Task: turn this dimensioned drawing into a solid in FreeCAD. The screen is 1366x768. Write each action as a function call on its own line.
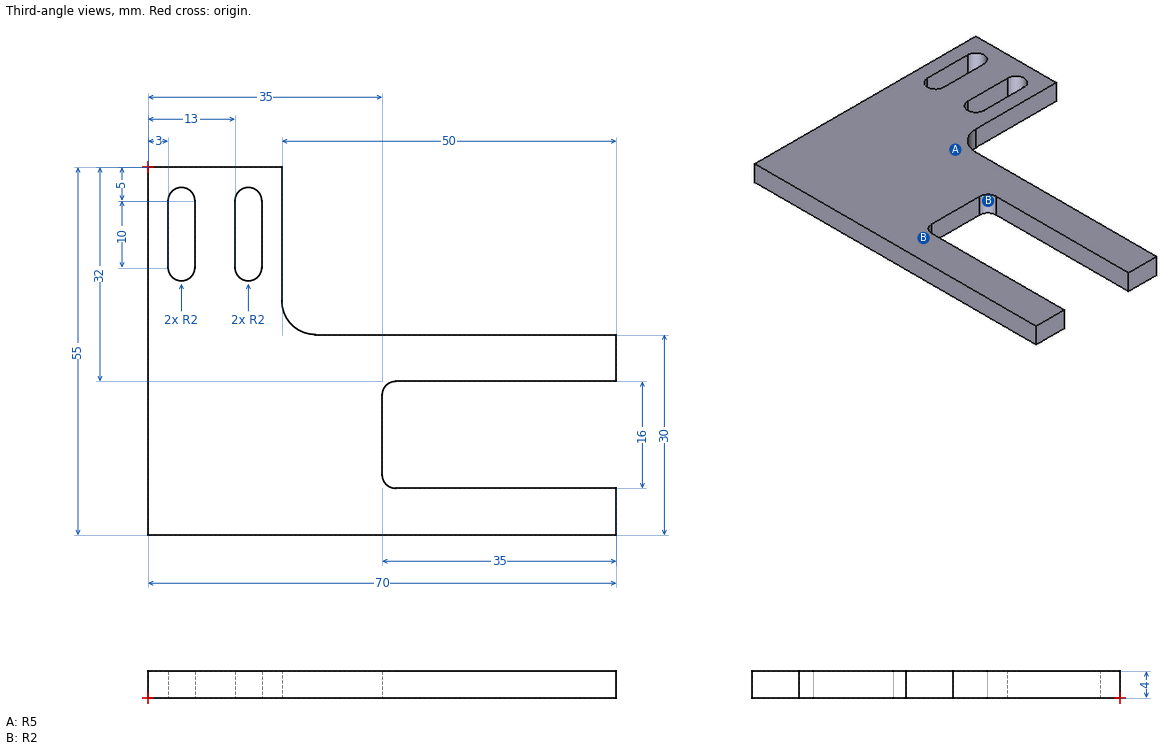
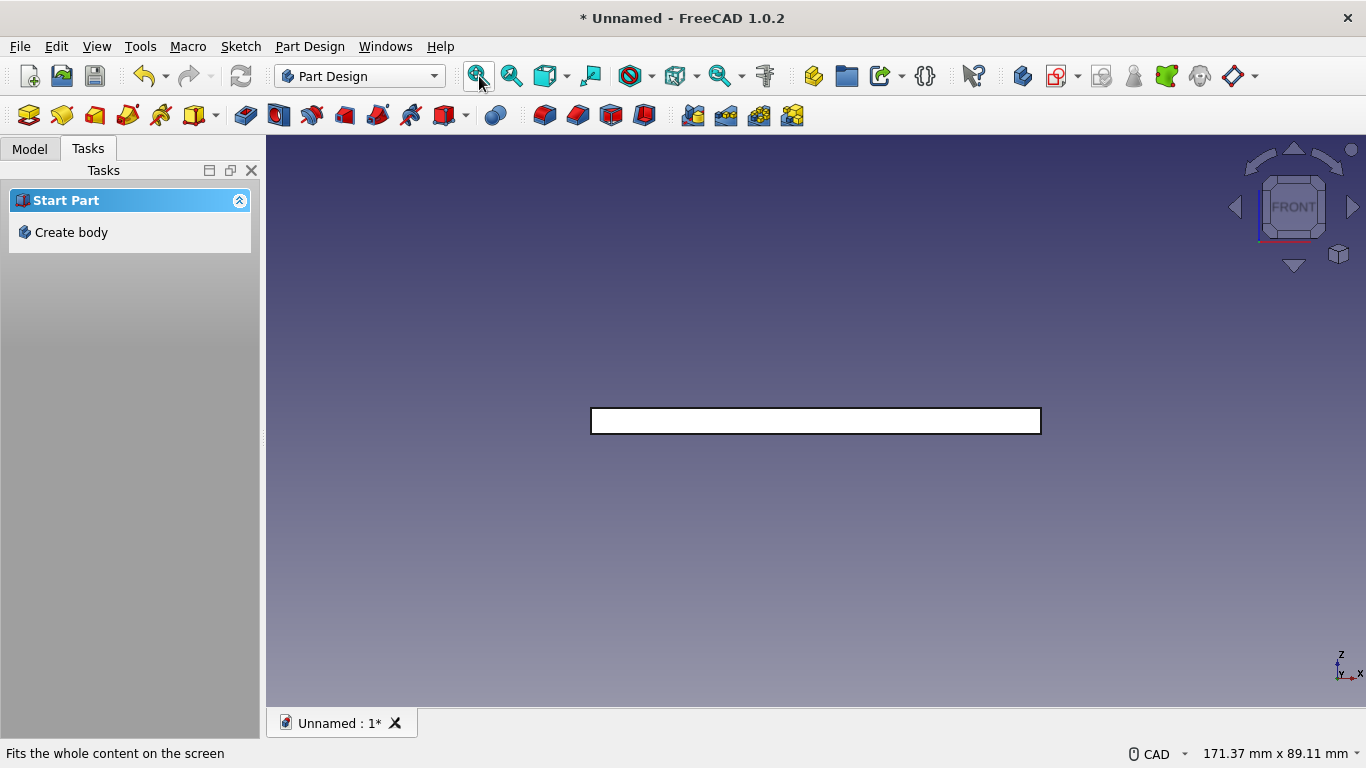
click(479, 76)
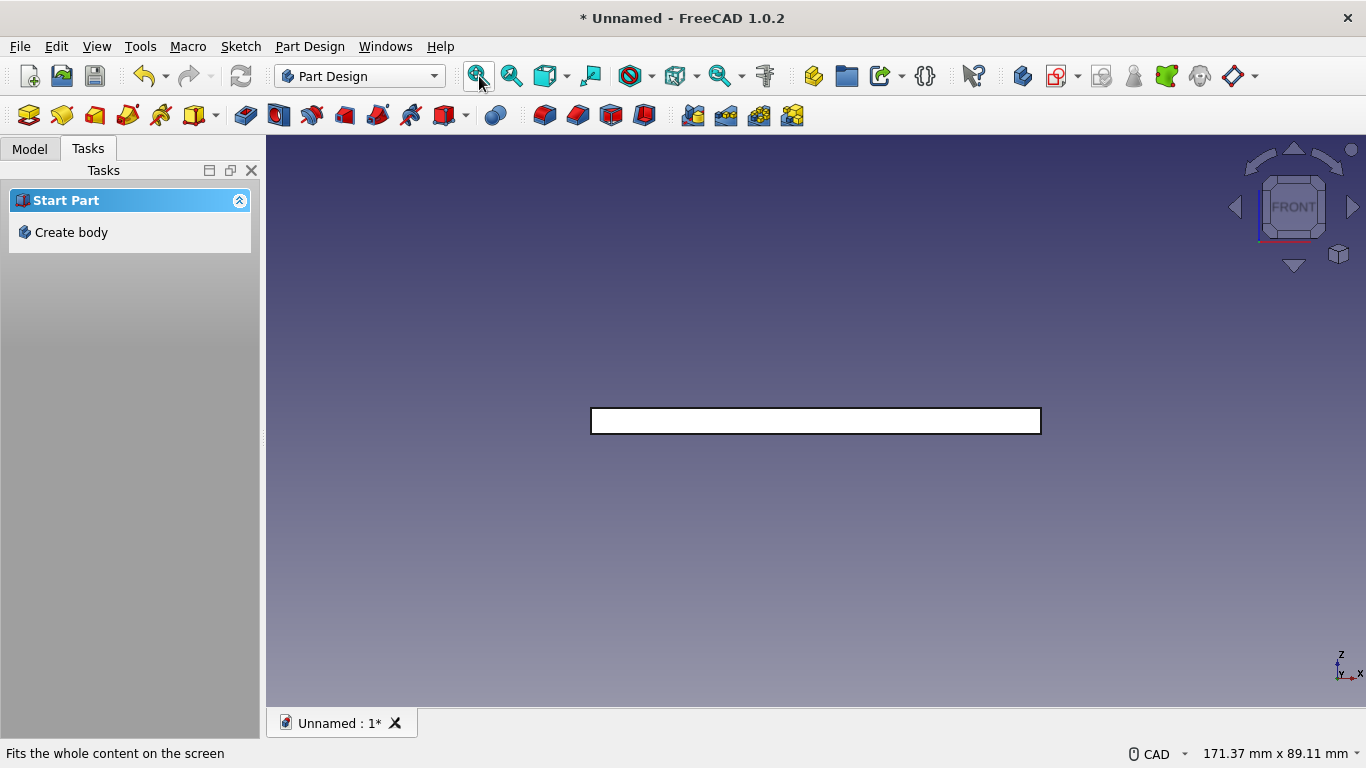
key(3)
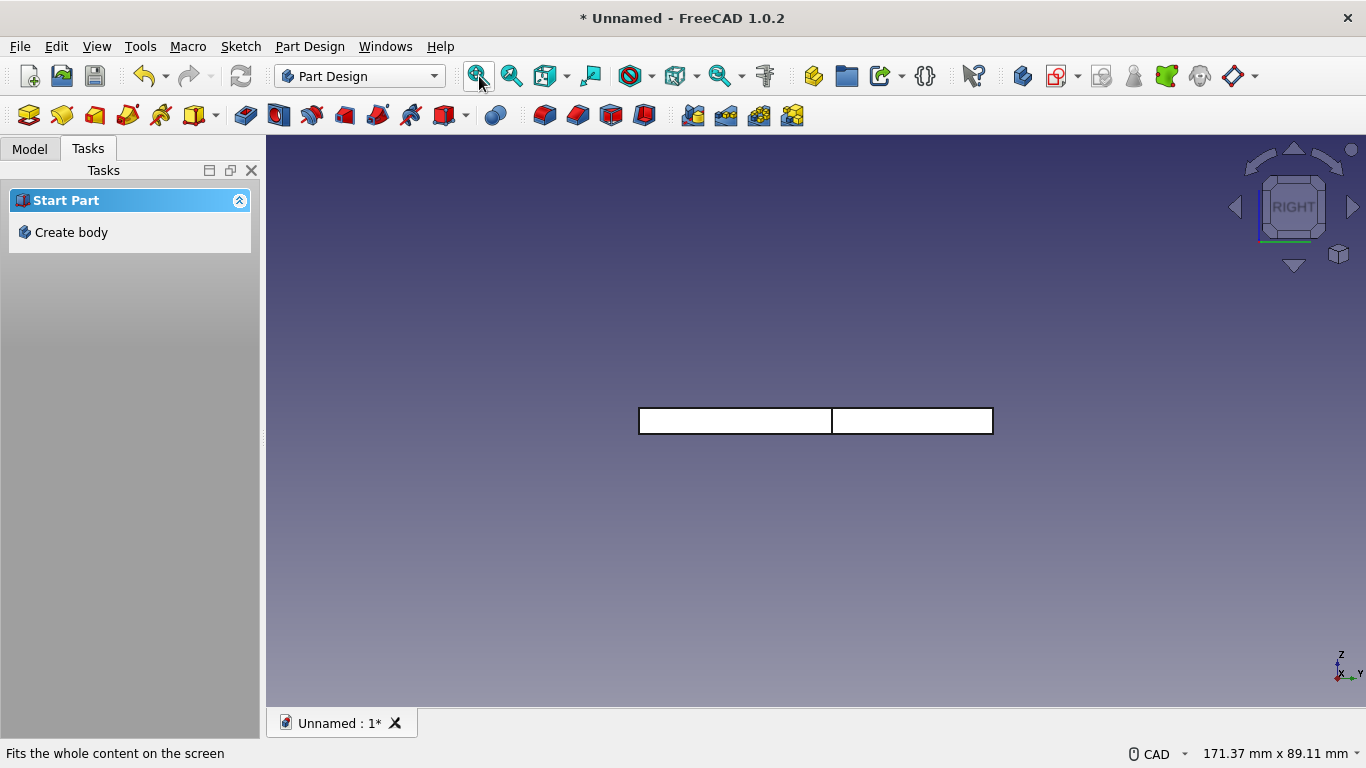
click(479, 76)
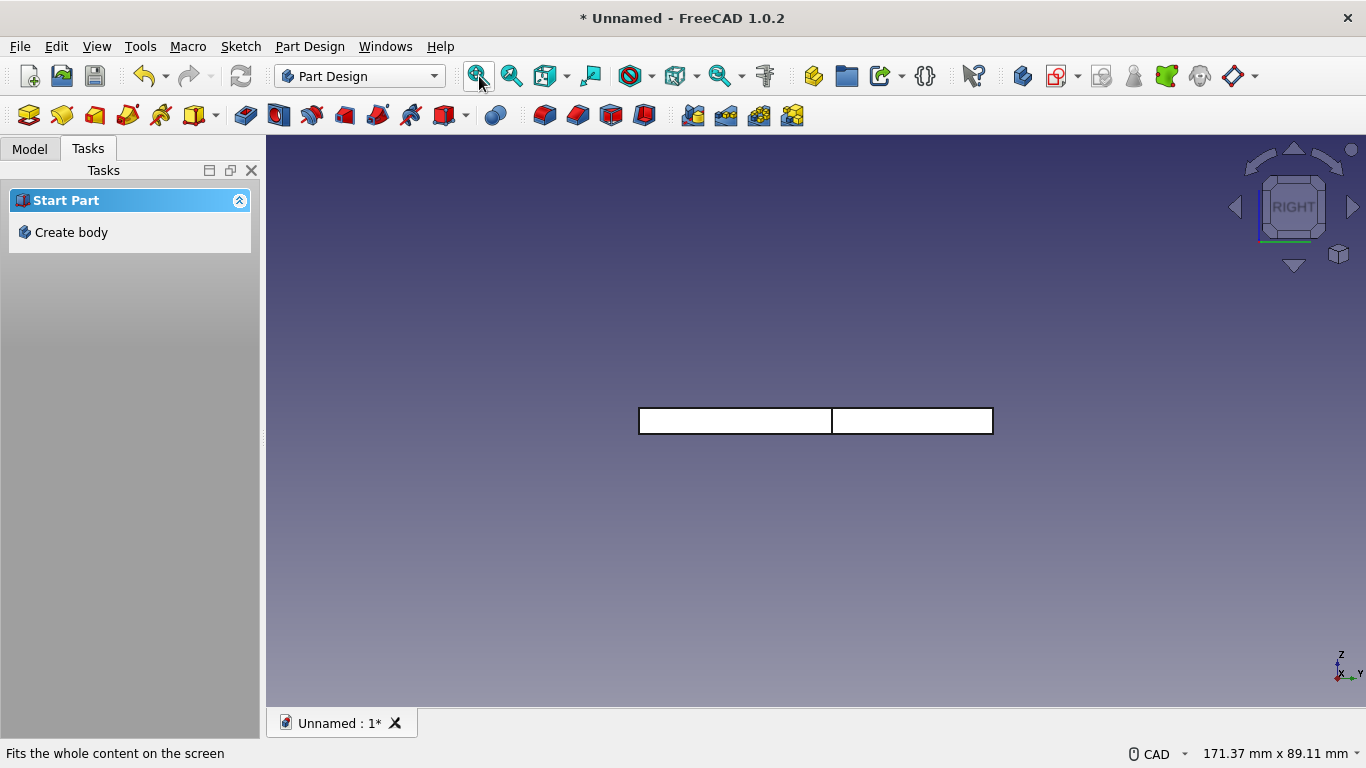
key(5)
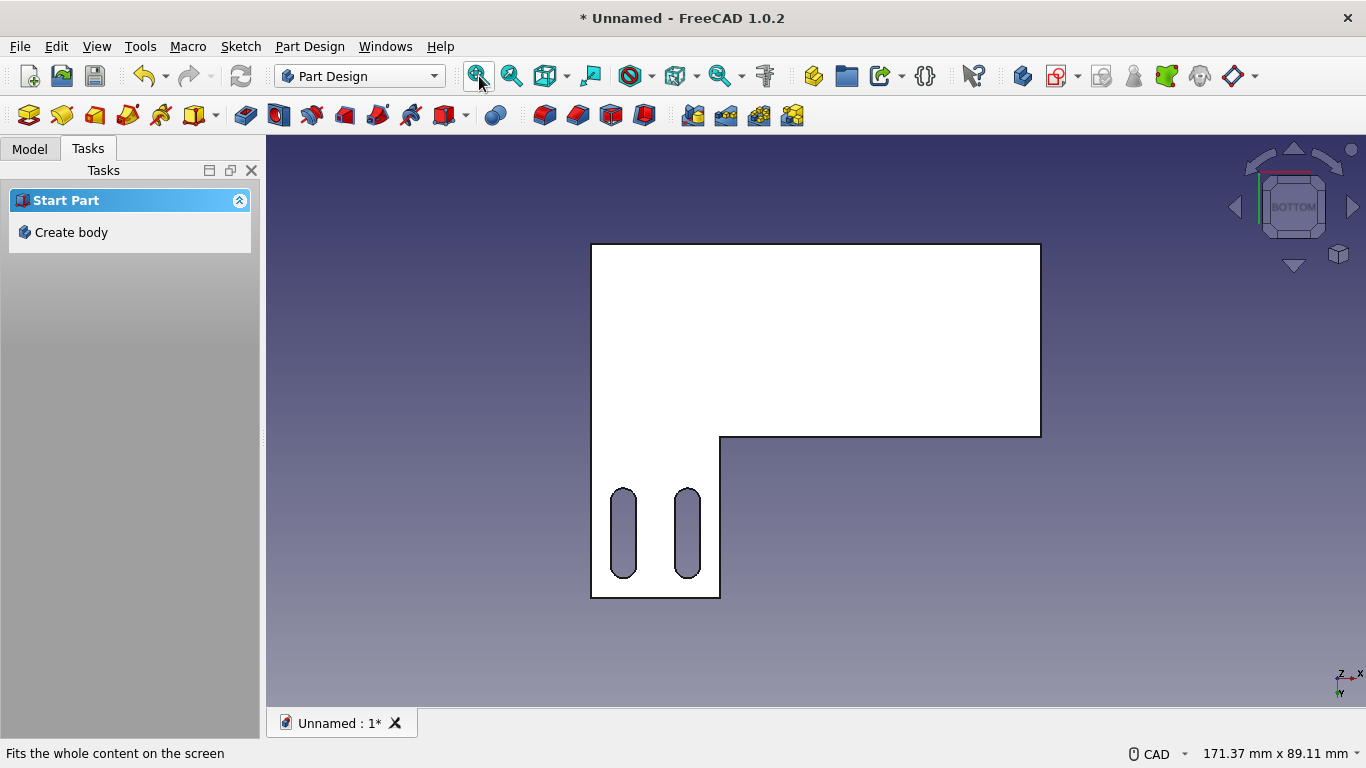
key(4)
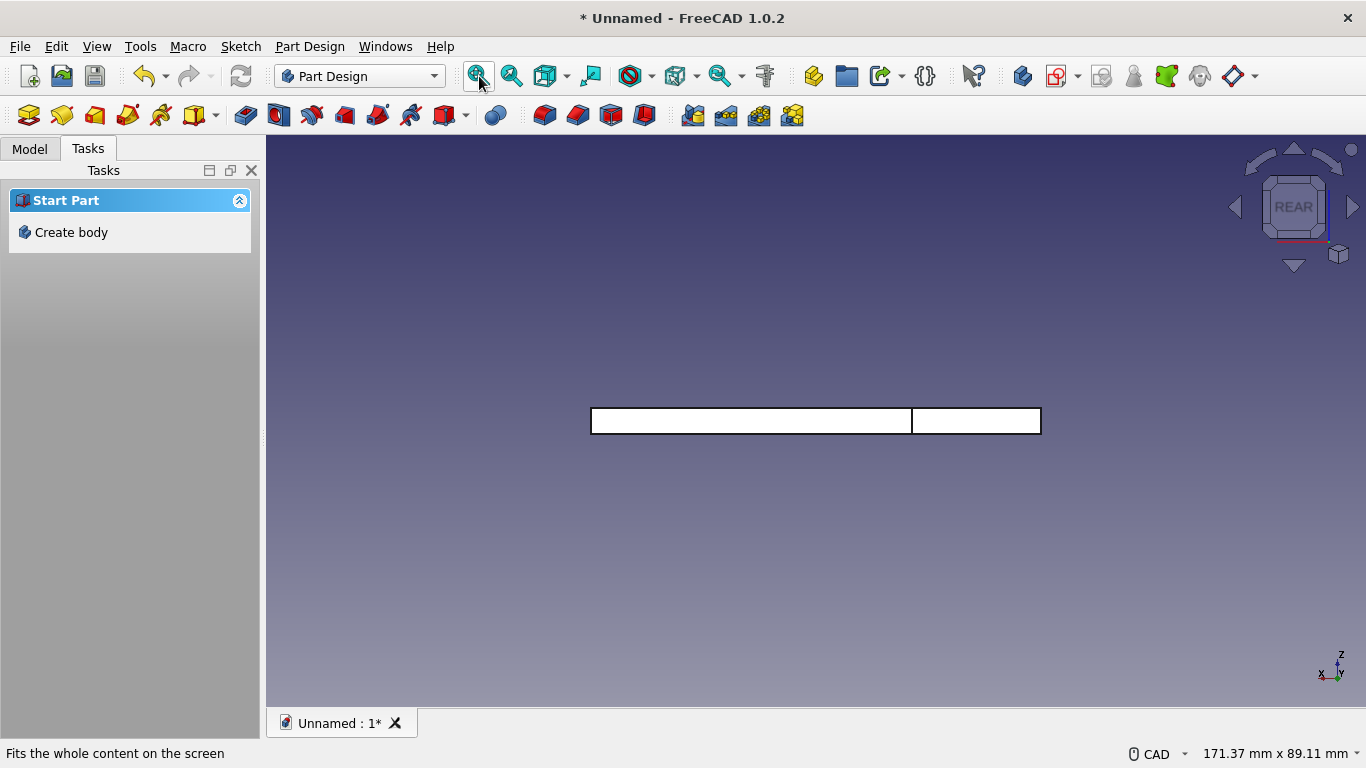
click(479, 76)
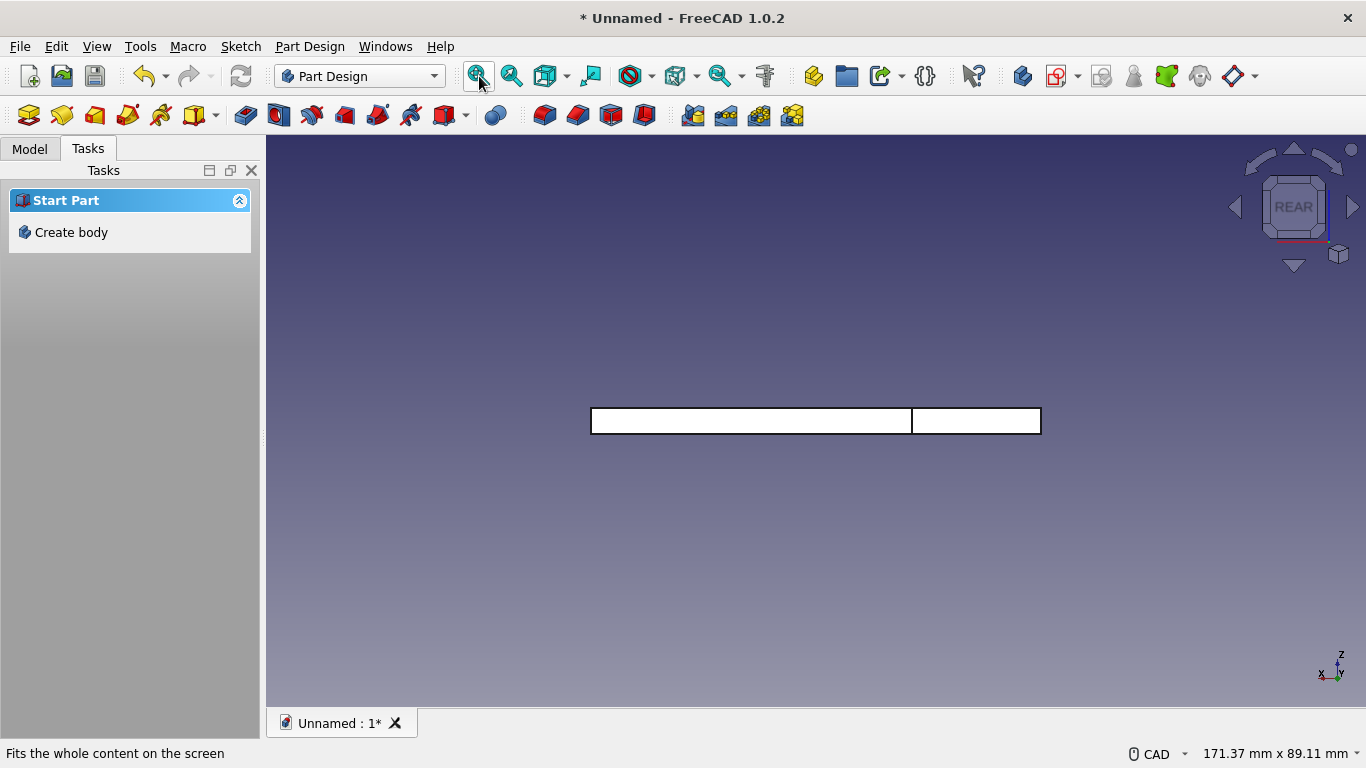
key(6)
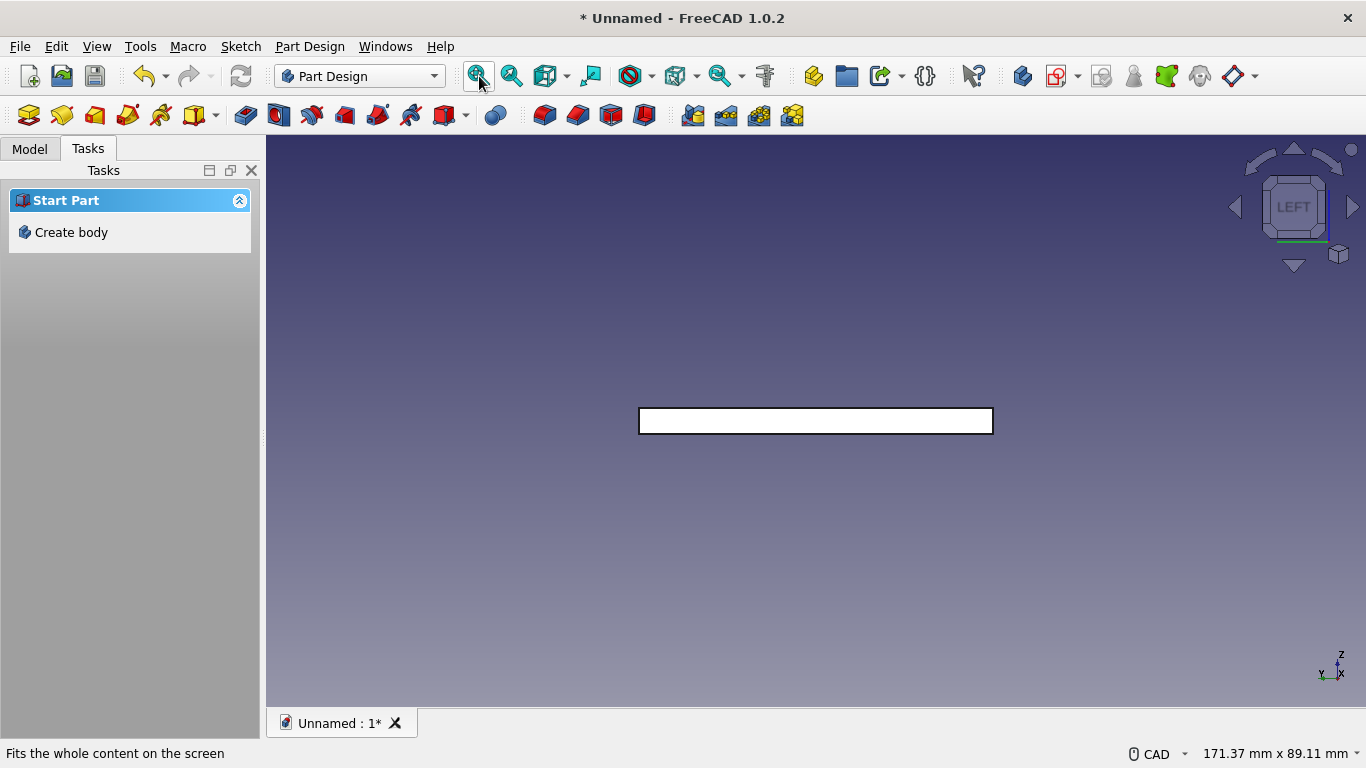
click(479, 76)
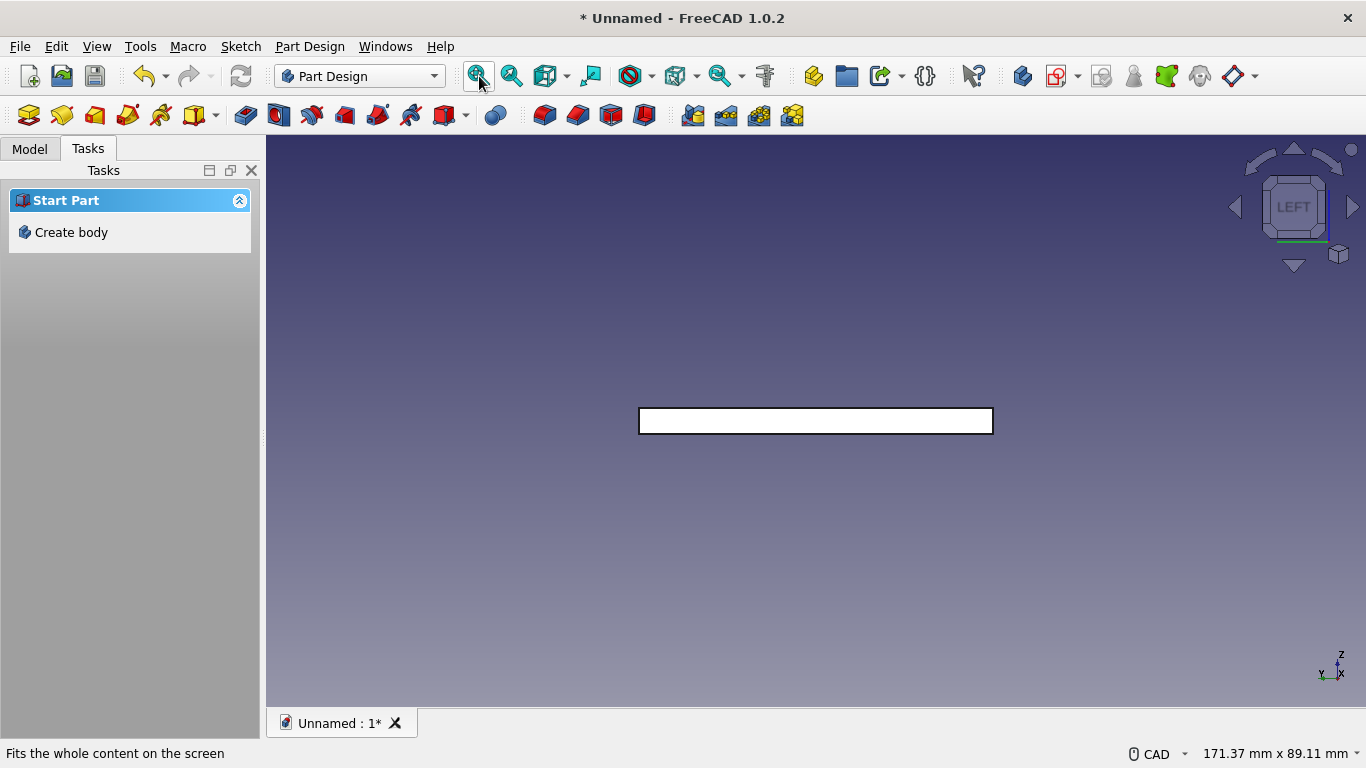
key(v)
key(3)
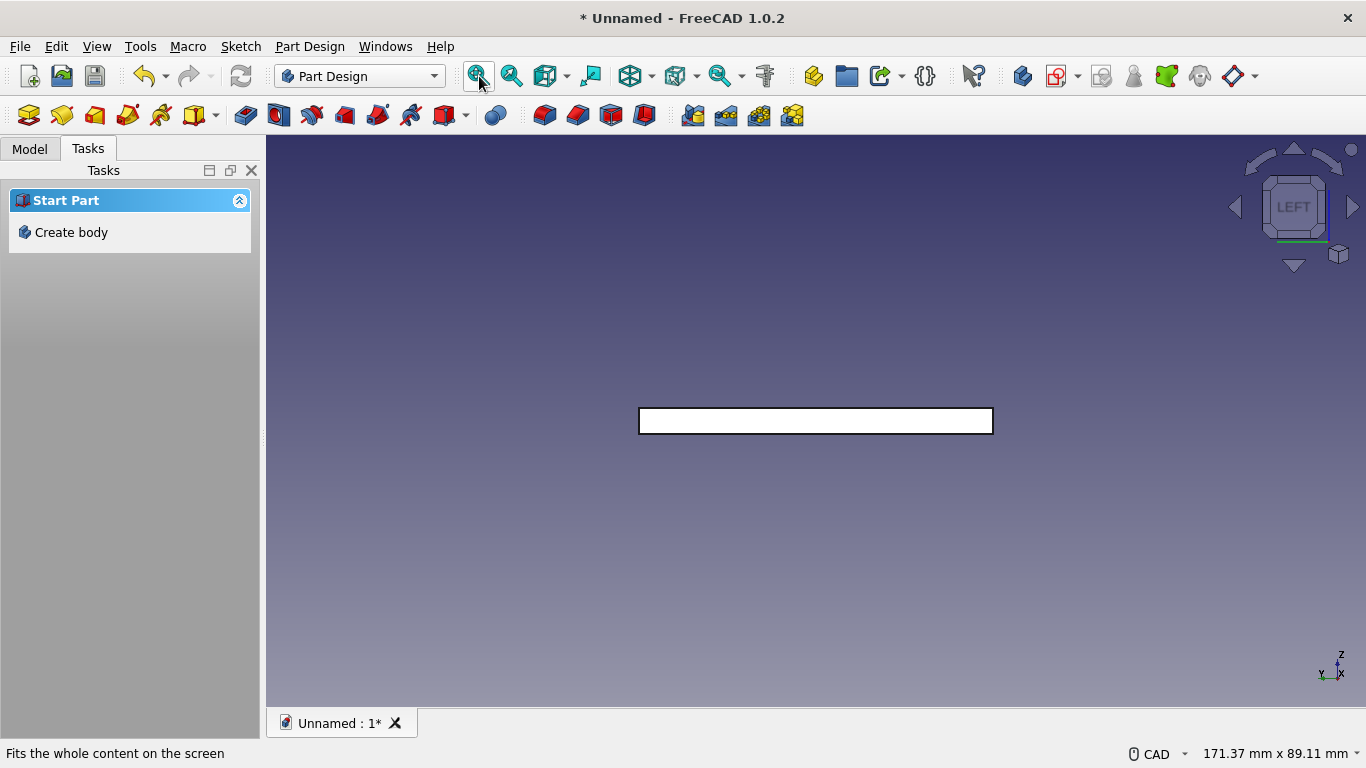
key(0)